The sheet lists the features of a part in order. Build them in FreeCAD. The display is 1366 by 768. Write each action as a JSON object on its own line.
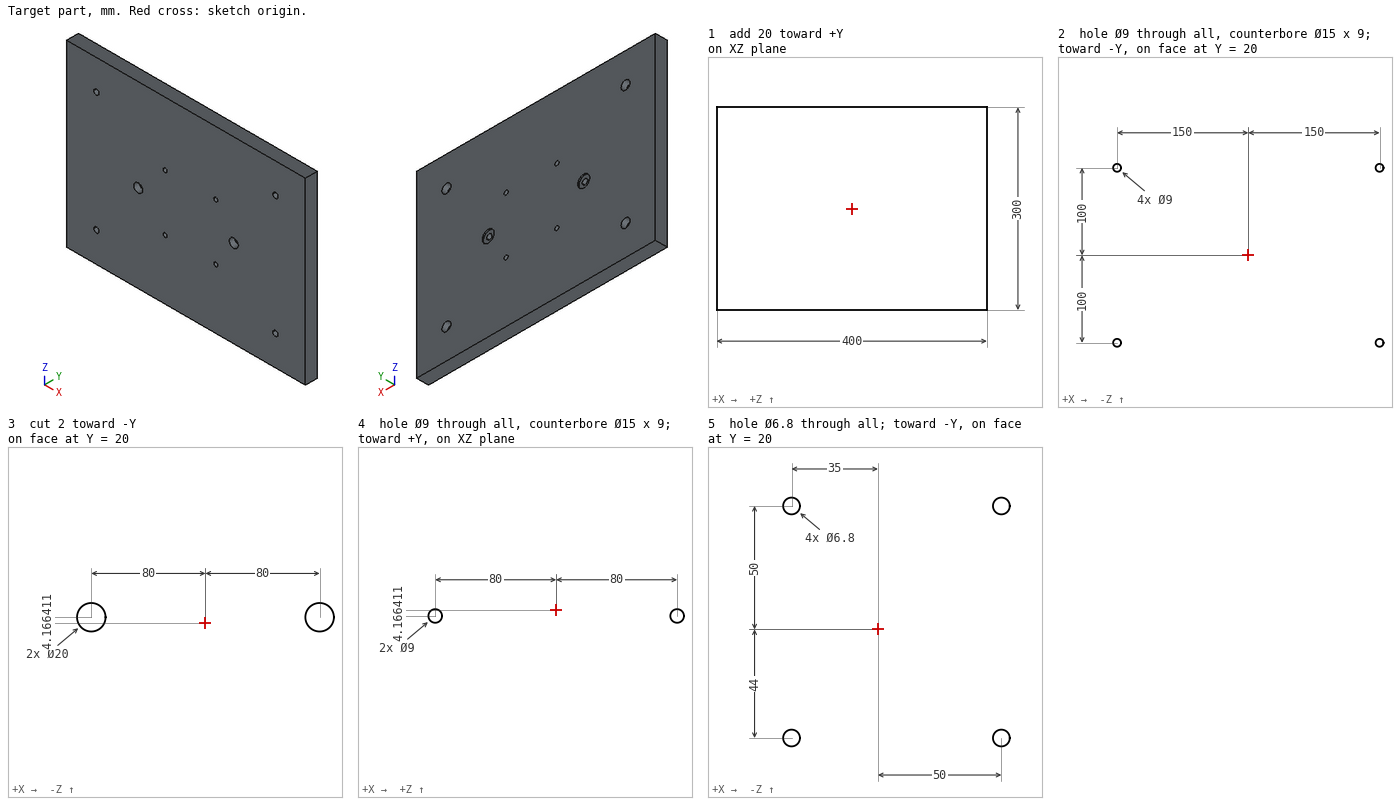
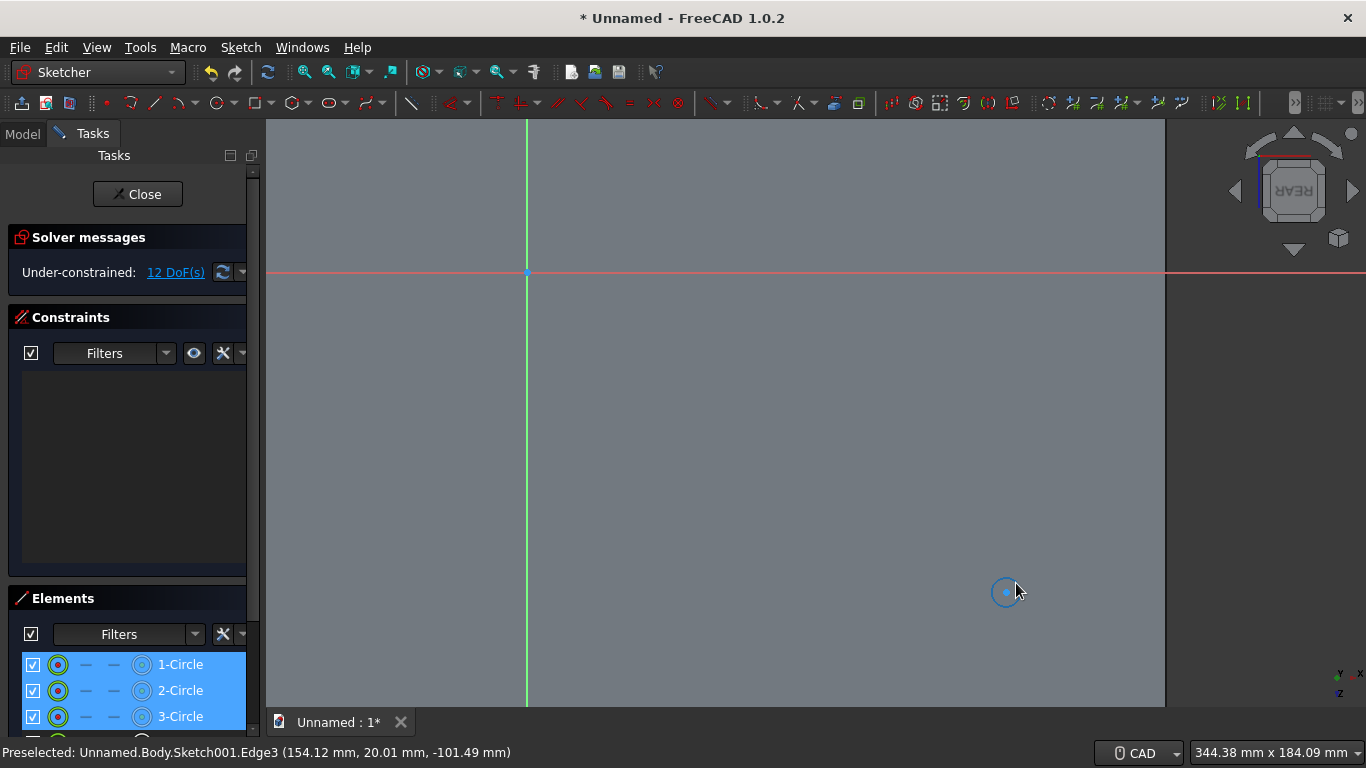
{"action": "left_click", "coordinate": [1016, 582]}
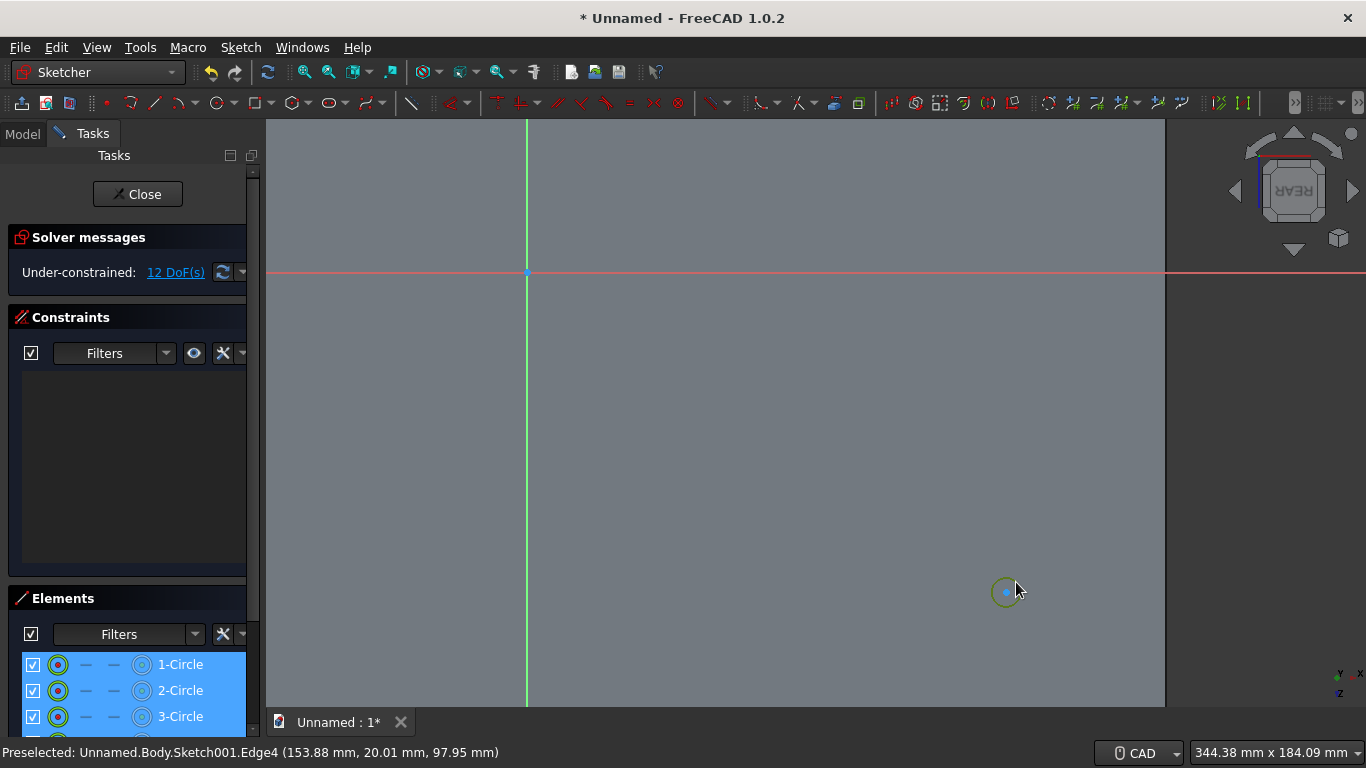
{"action": "key", "text": "e"}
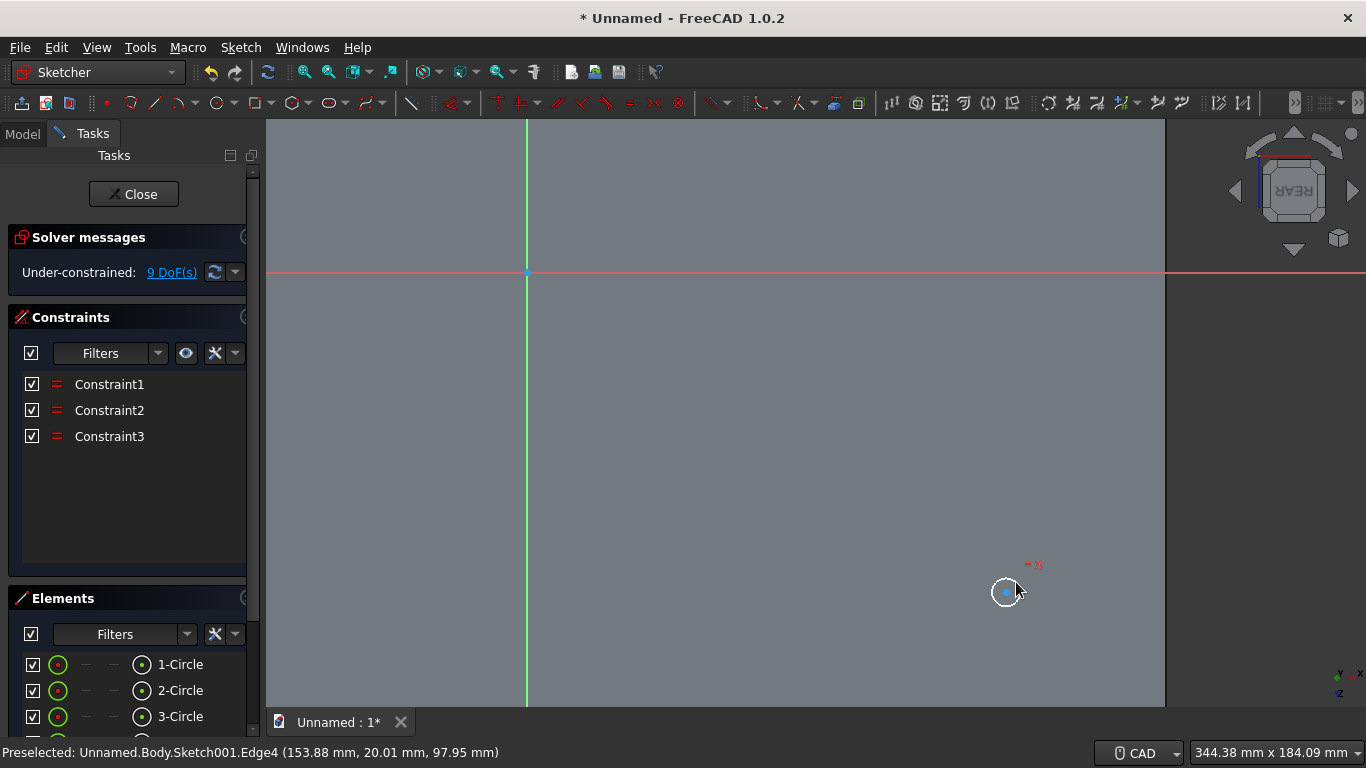
{"action": "scroll", "coordinate": [1016, 584], "scroll_direction": "down", "scroll_amount": 3}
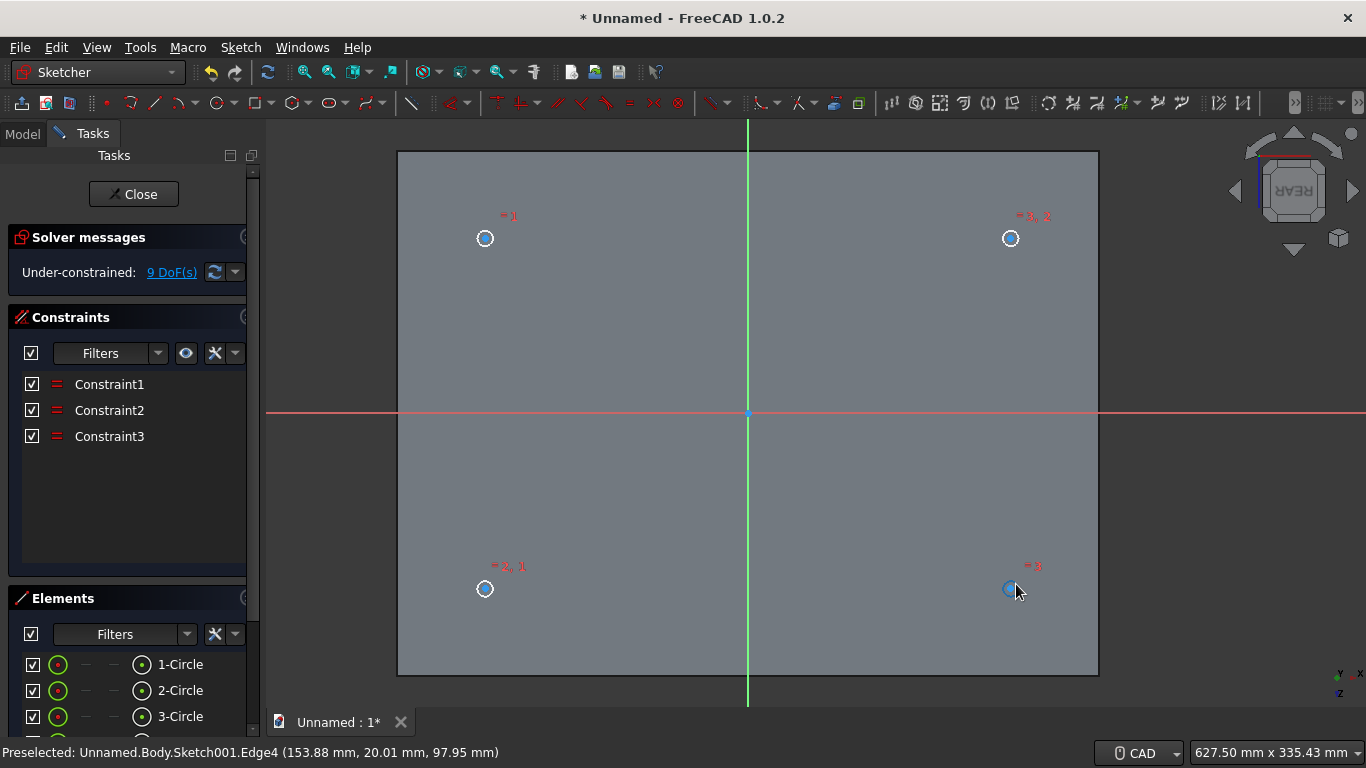
{"action": "left_click", "coordinate": [485, 238]}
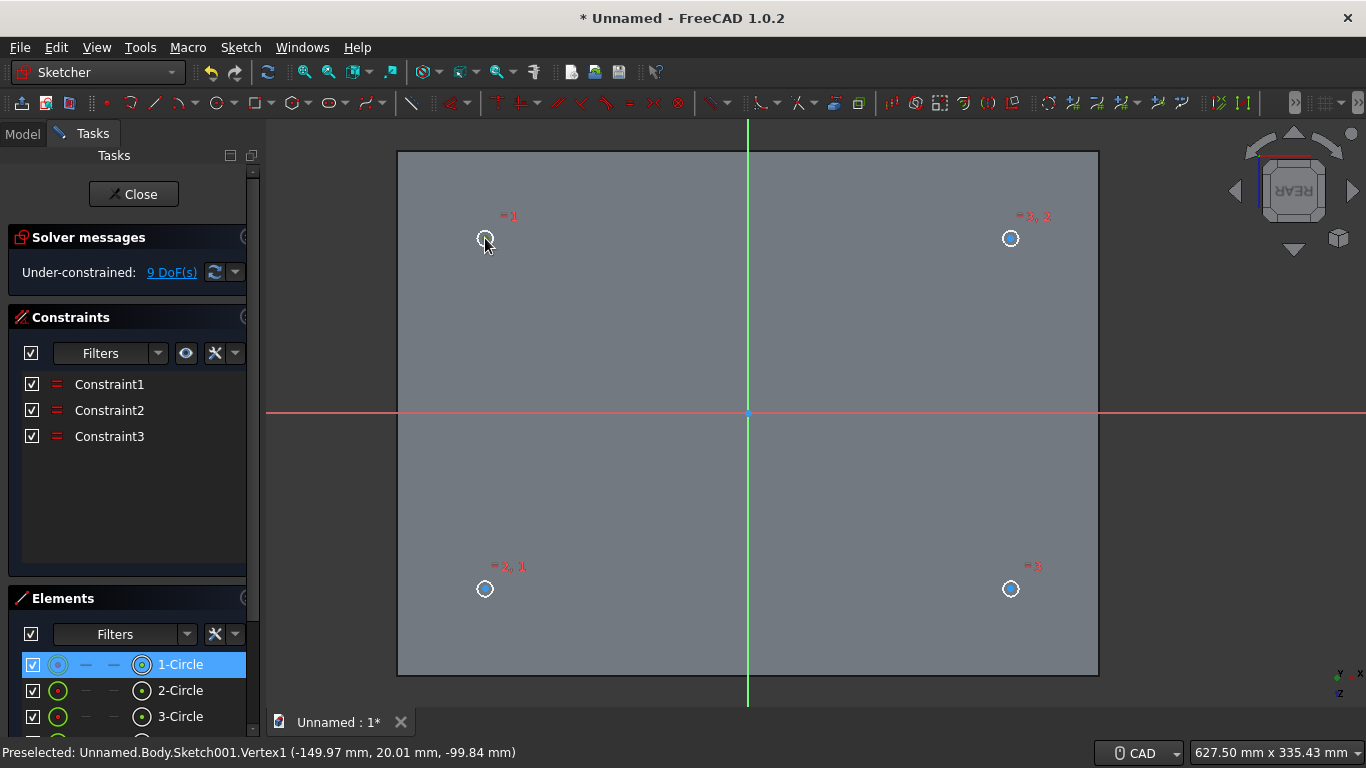
{"action": "left_click", "coordinate": [485, 589]}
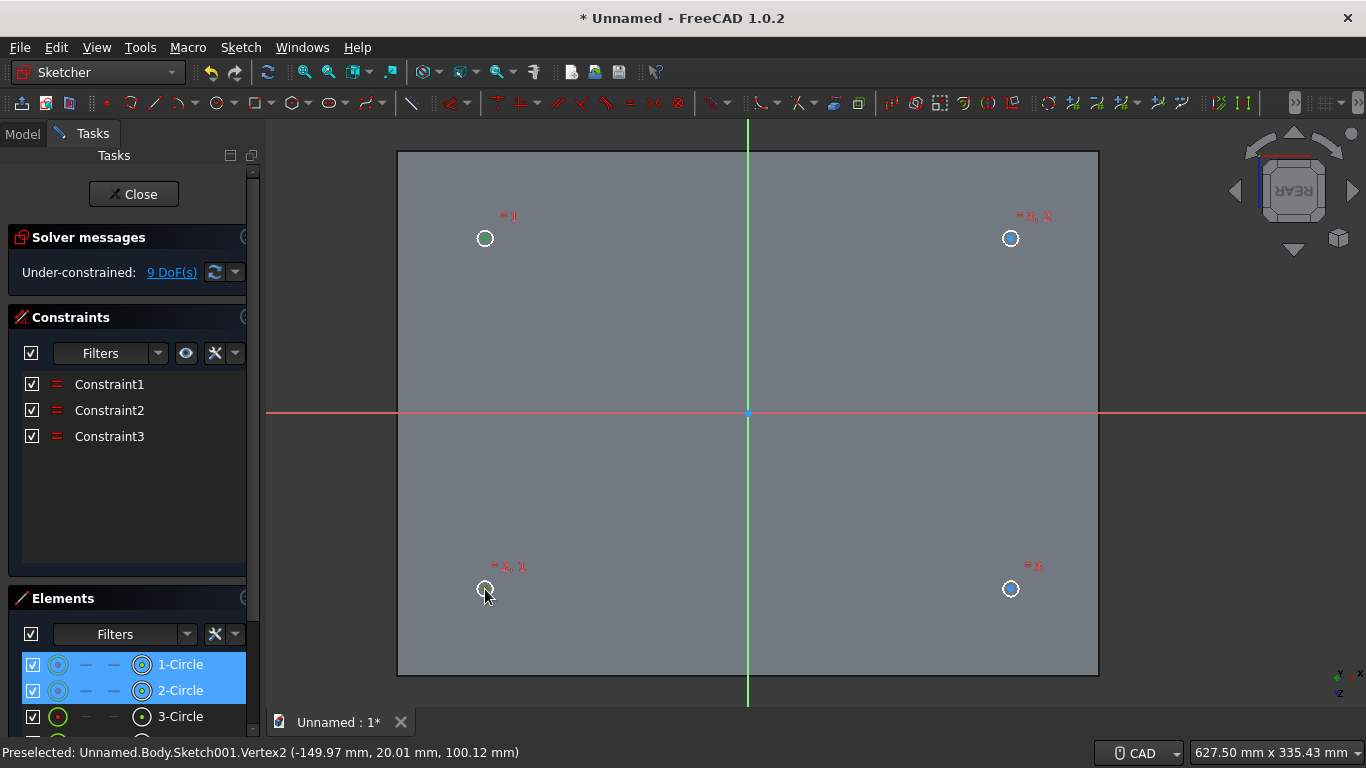
{"action": "key", "text": "v"}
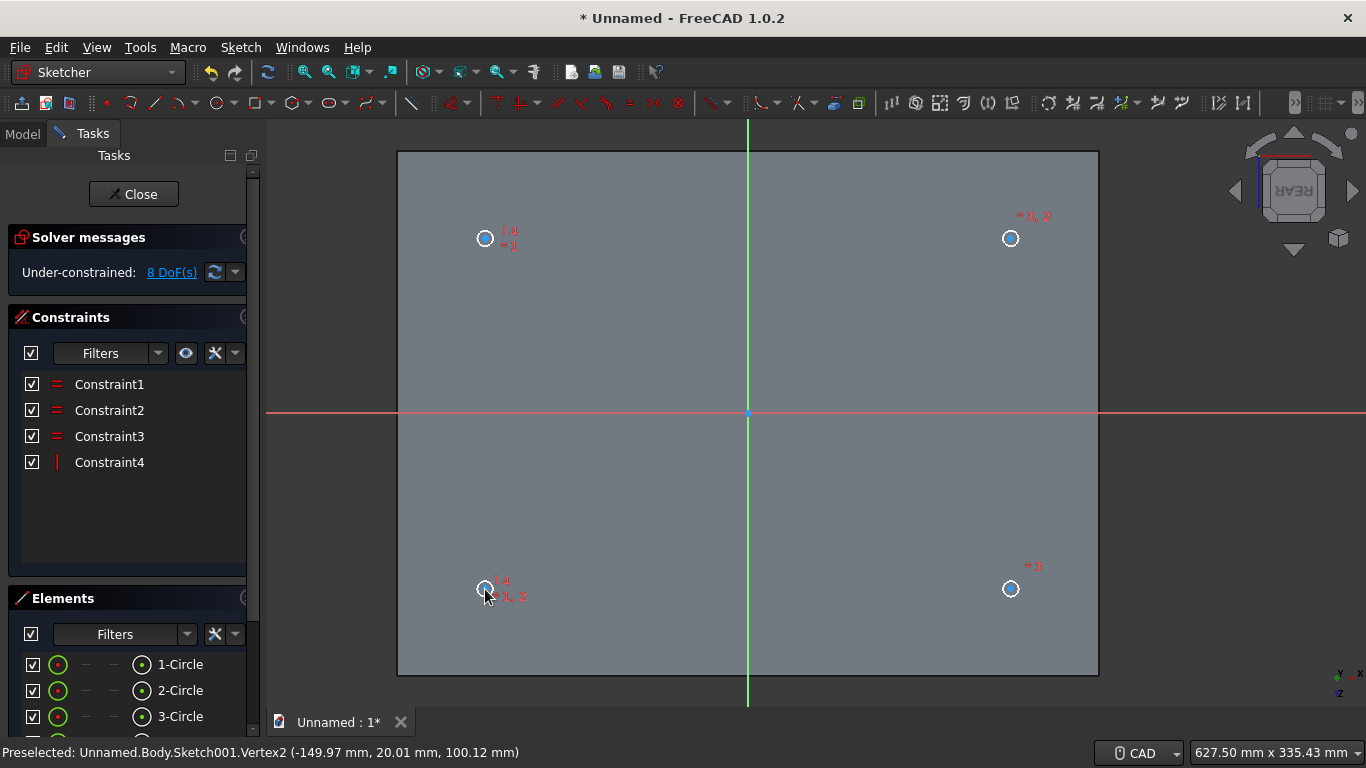
{"action": "left_click", "coordinate": [485, 238]}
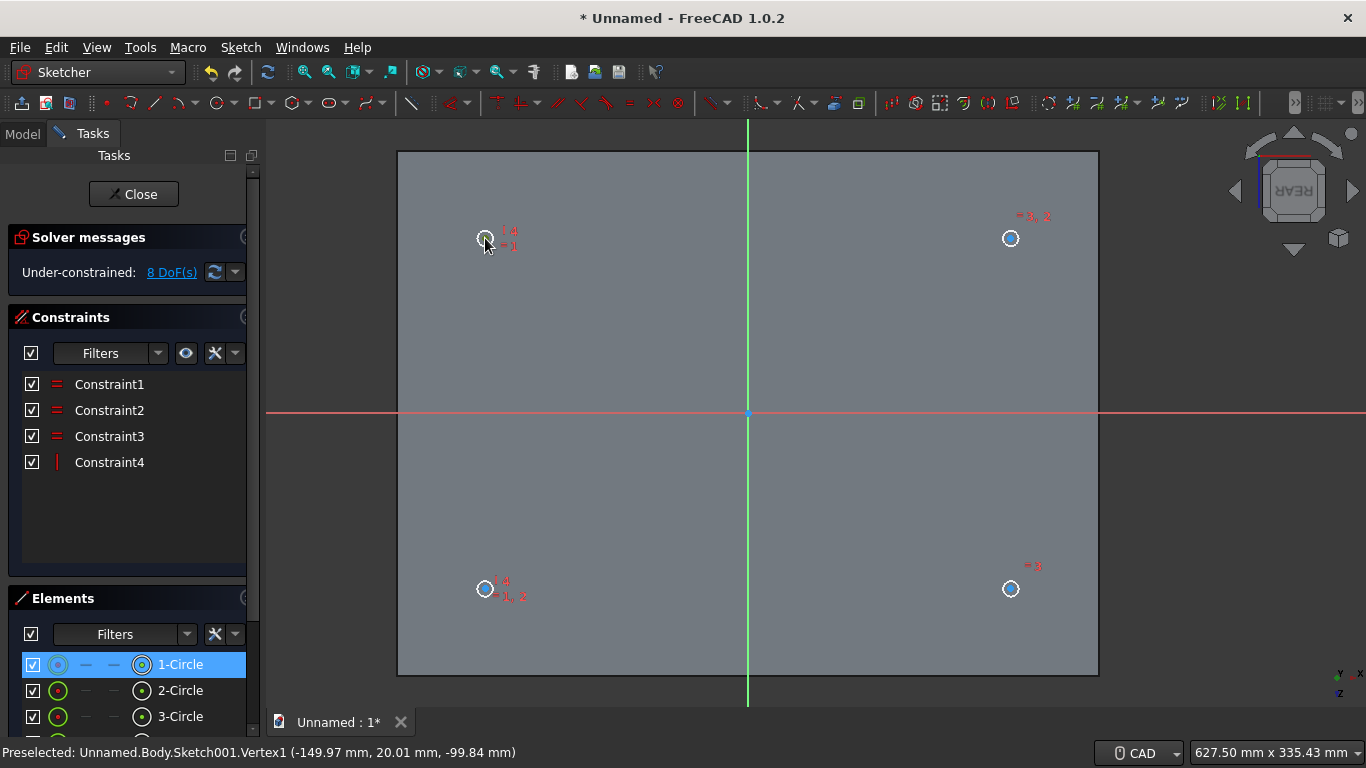
{"action": "left_click", "coordinate": [1011, 238]}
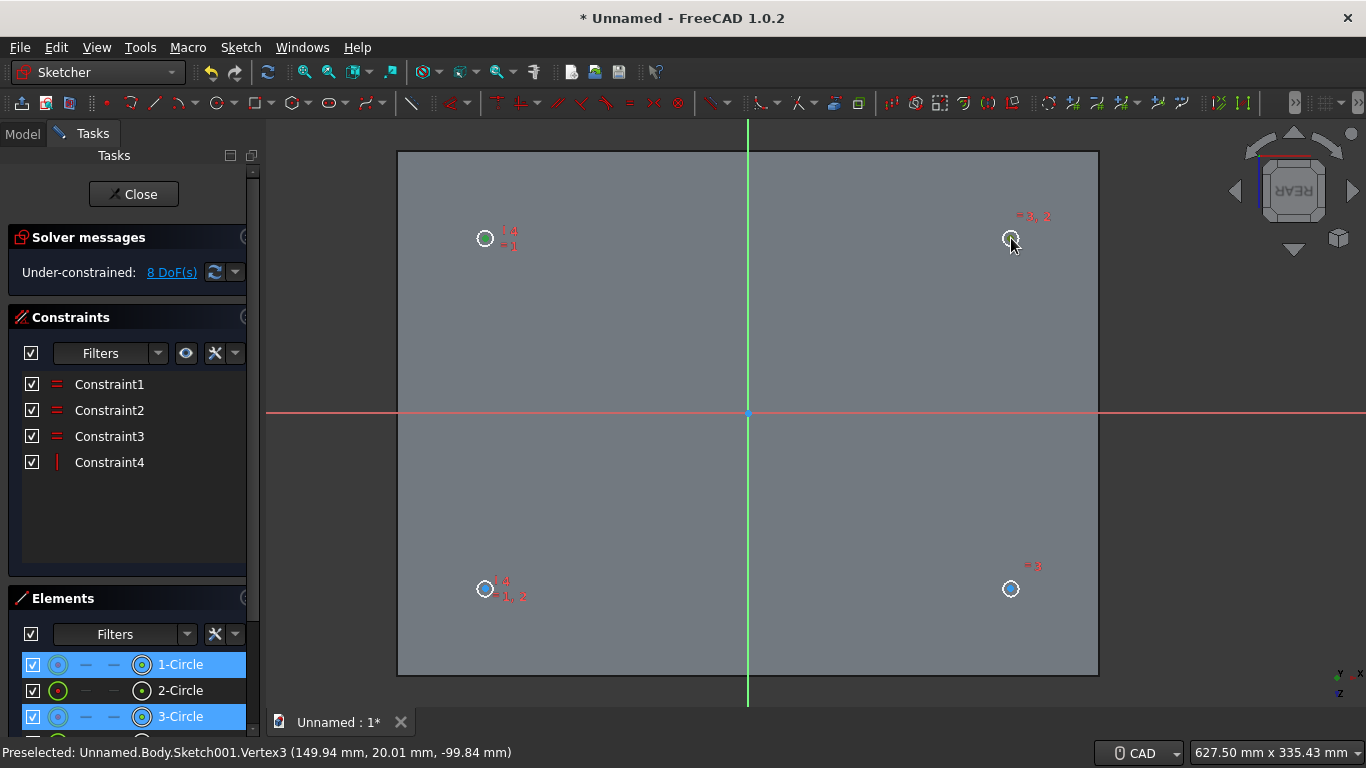
{"action": "key", "text": "h"}